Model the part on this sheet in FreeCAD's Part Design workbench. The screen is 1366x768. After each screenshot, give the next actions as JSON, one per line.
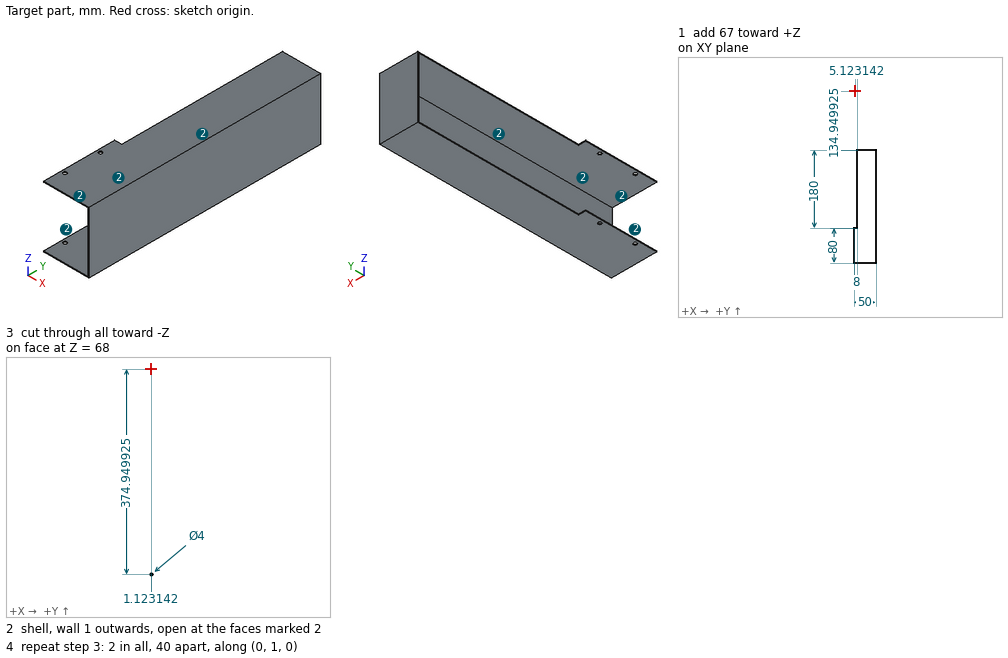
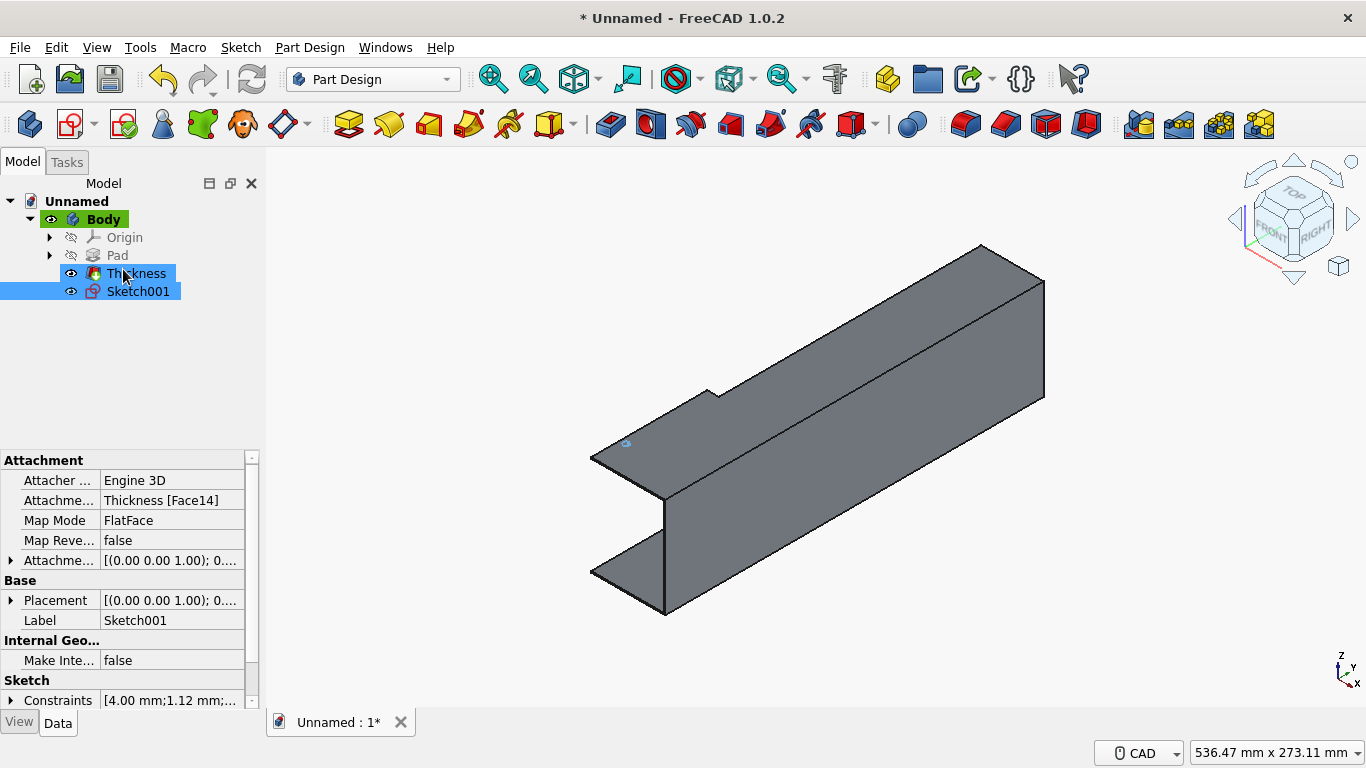
{"action": "left_click", "coordinate": [612, 124]}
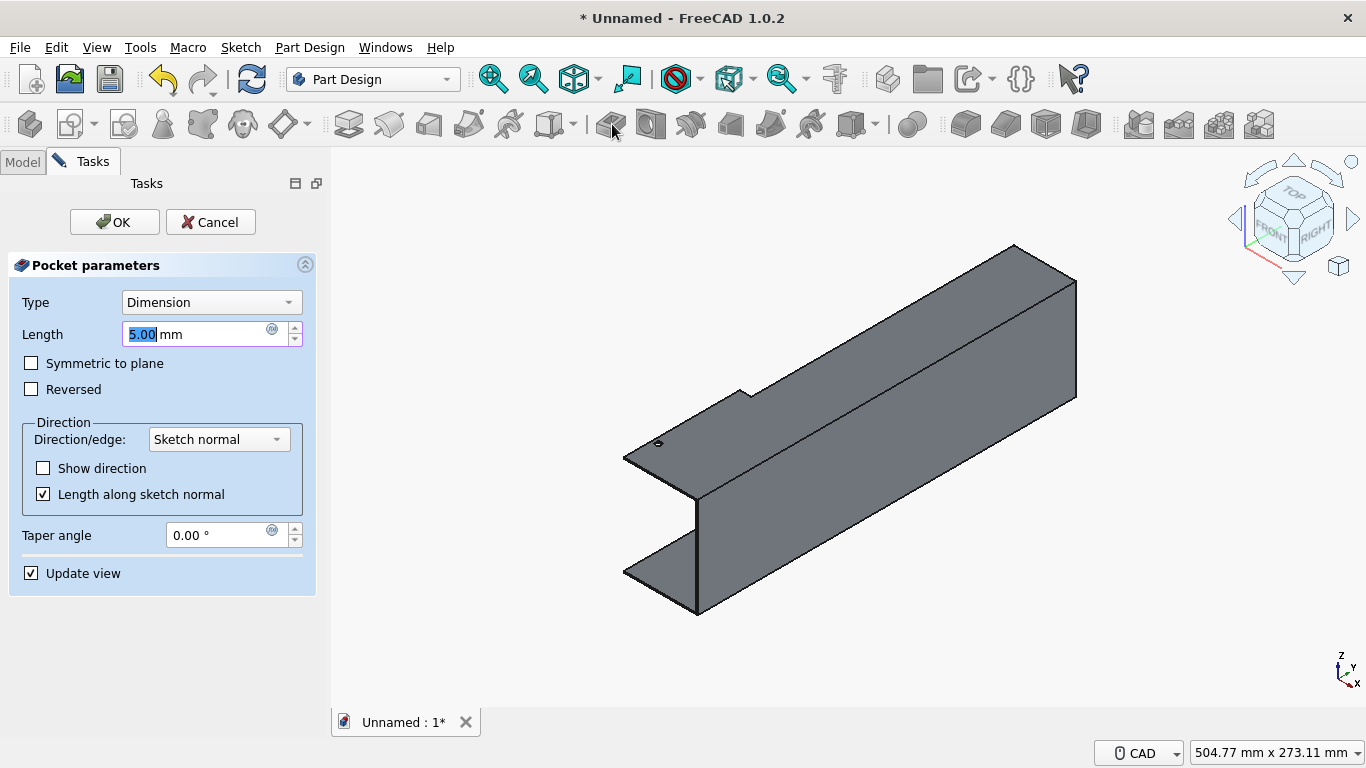
{"action": "left_click", "coordinate": [212, 302]}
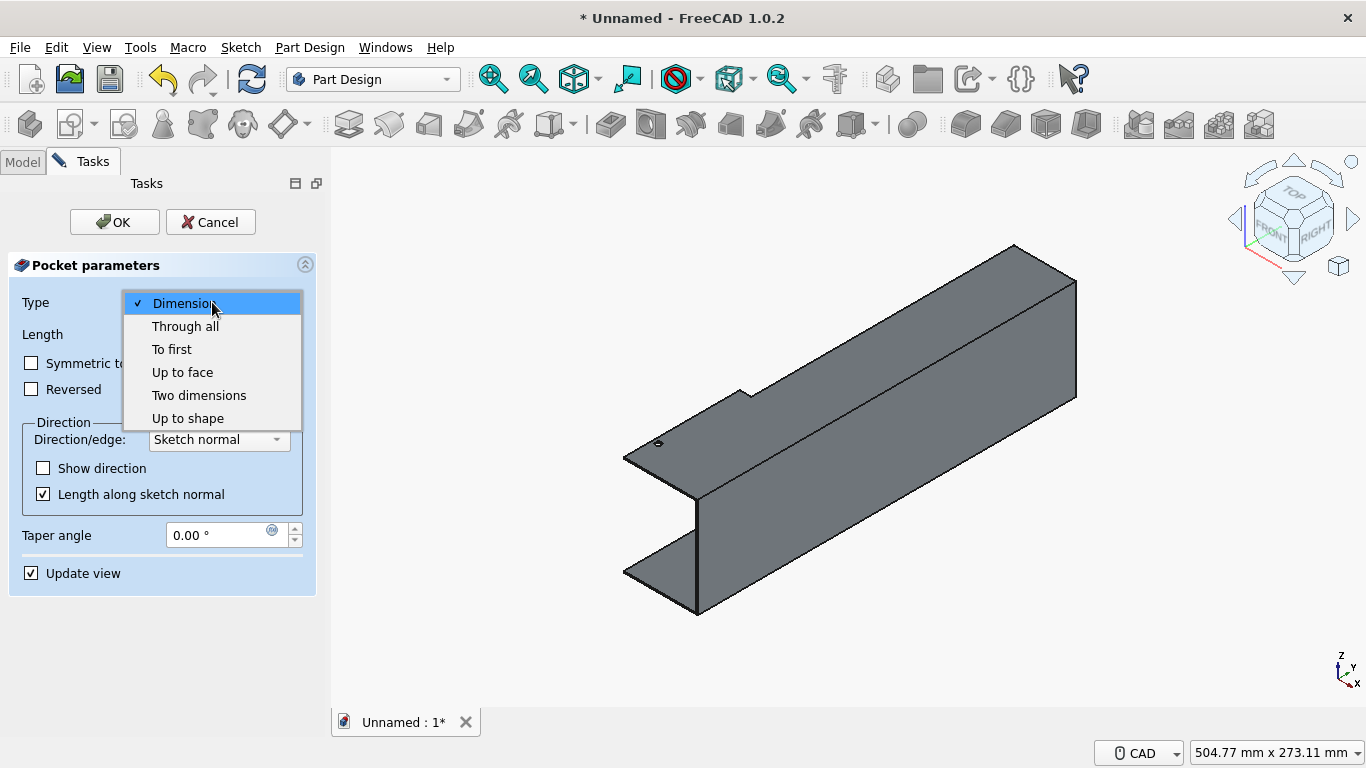
{"action": "left_click", "coordinate": [212, 326]}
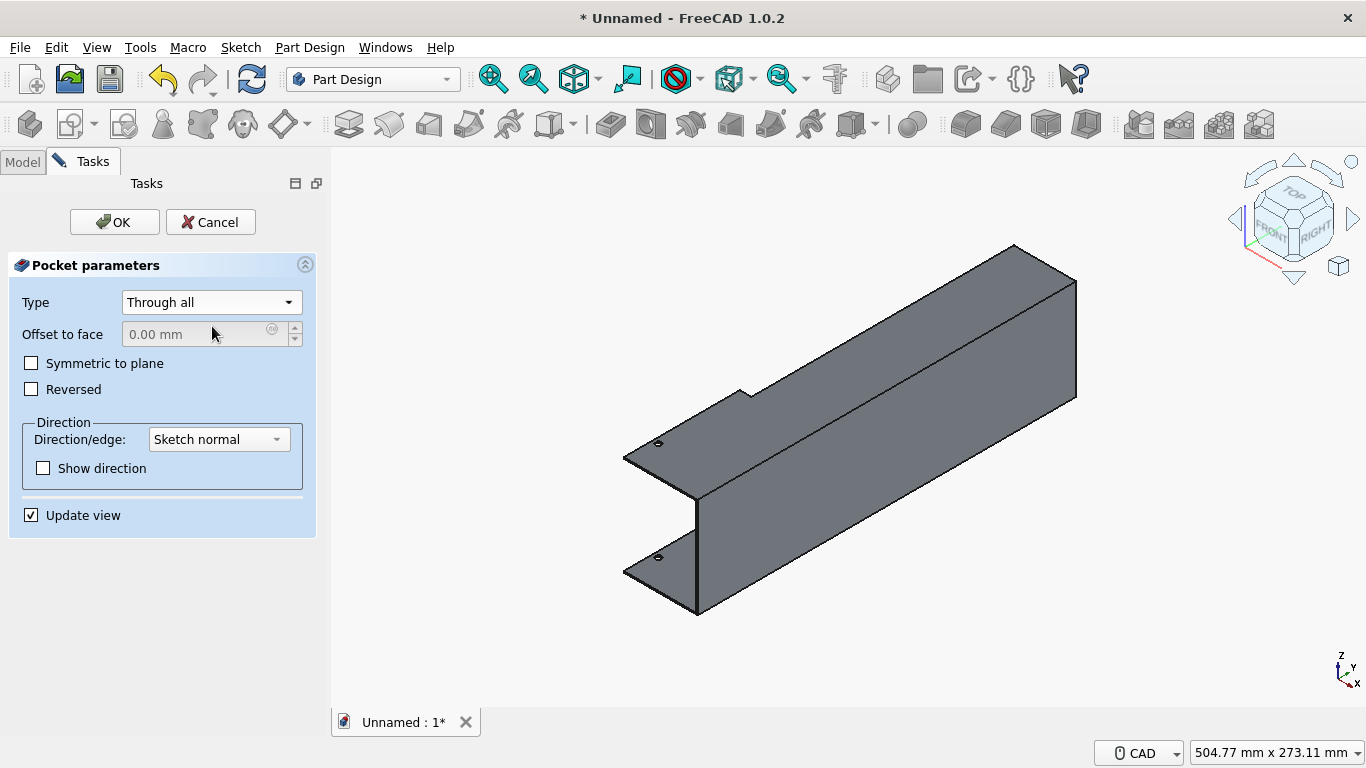
{"action": "left_click", "coordinate": [115, 222]}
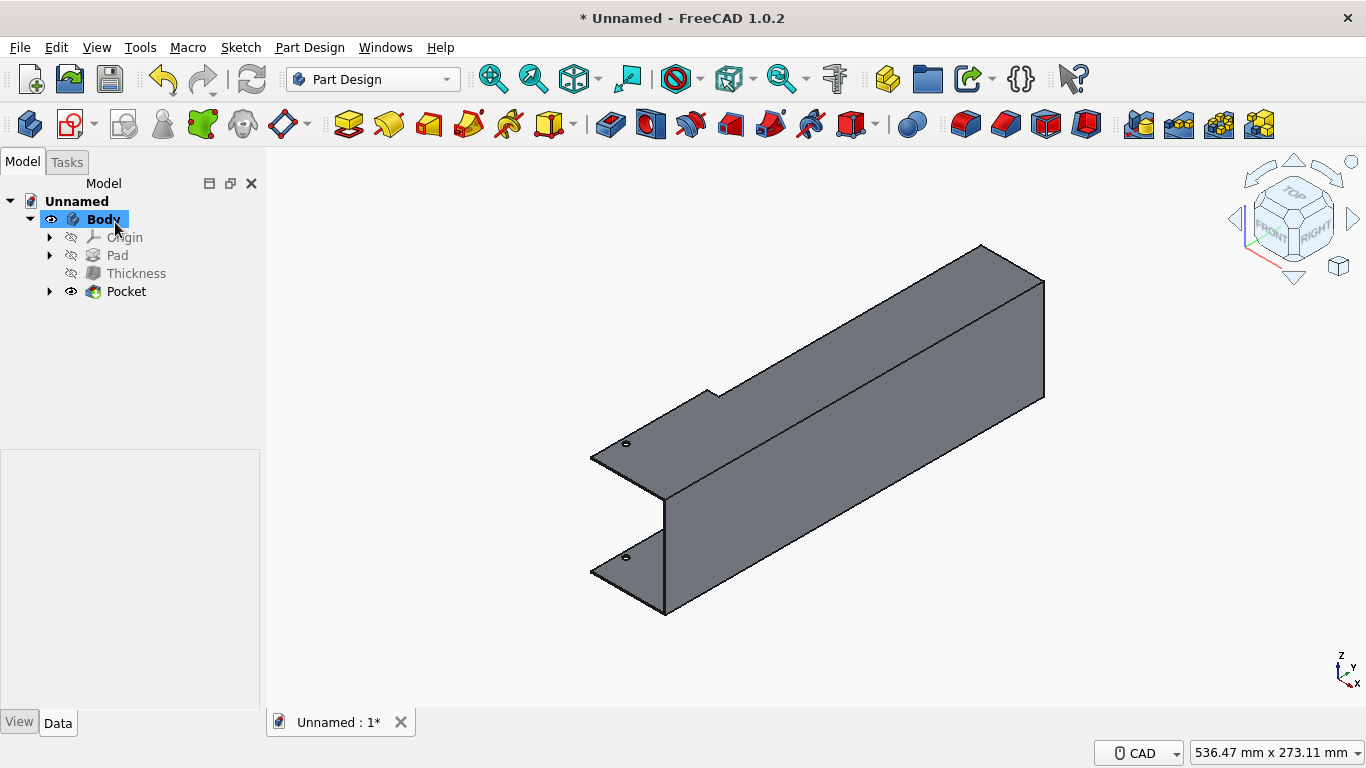
{"action": "left_click", "coordinate": [116, 291]}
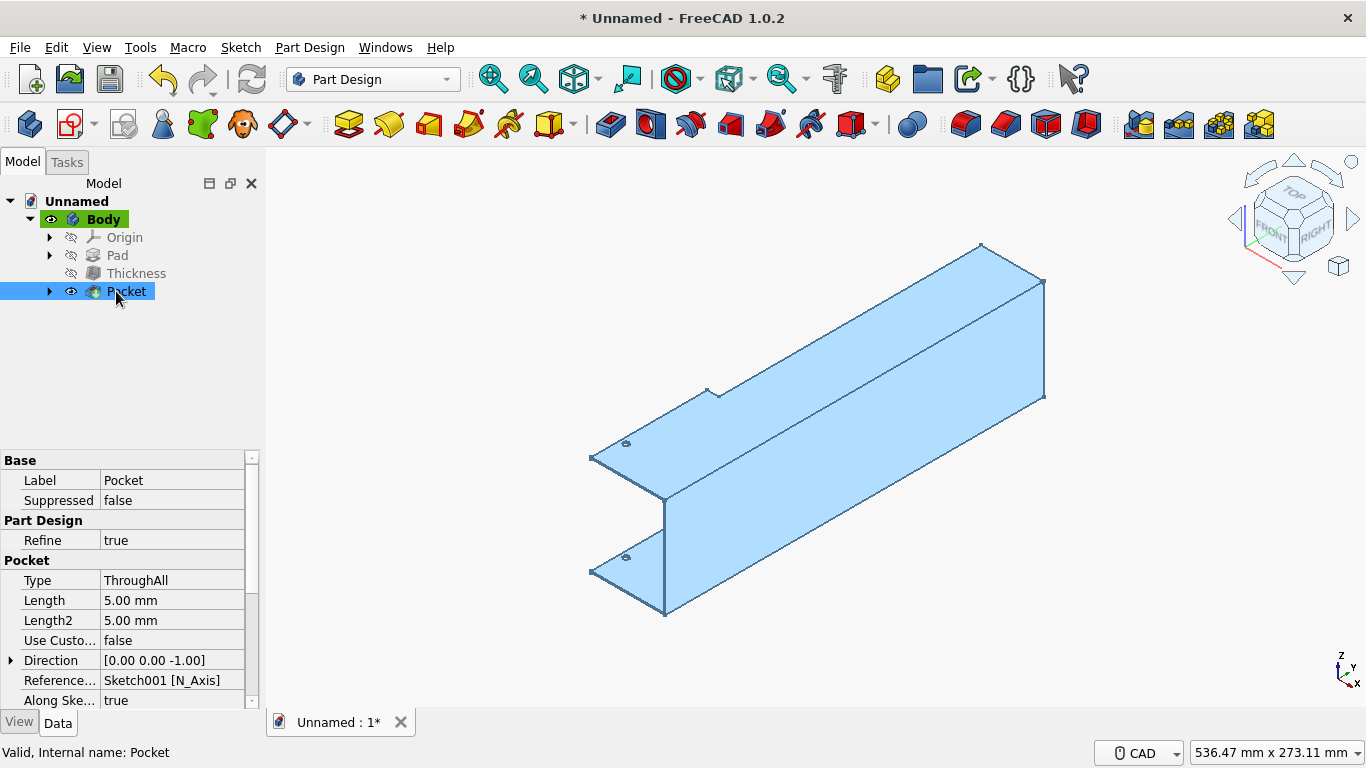
{"action": "left_click", "coordinate": [1180, 124]}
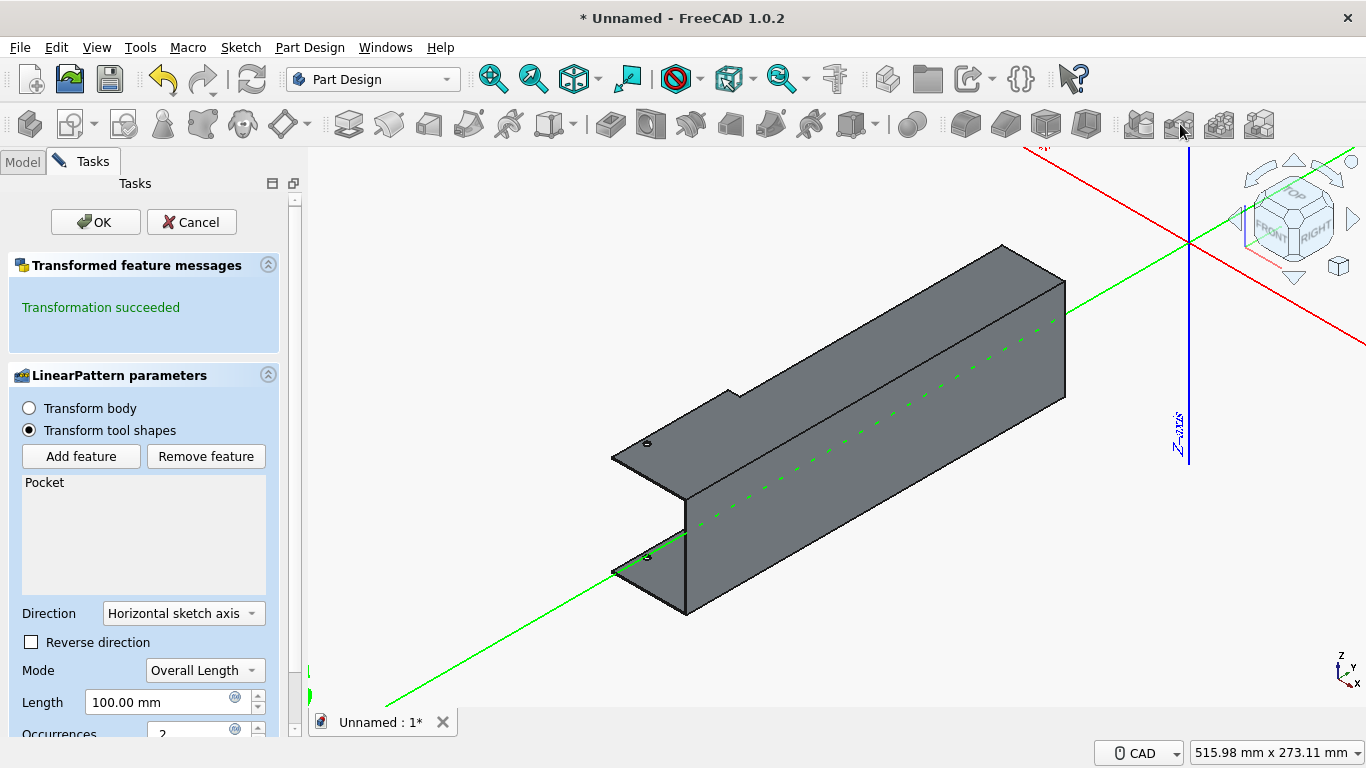
{"action": "left_click", "coordinate": [184, 614]}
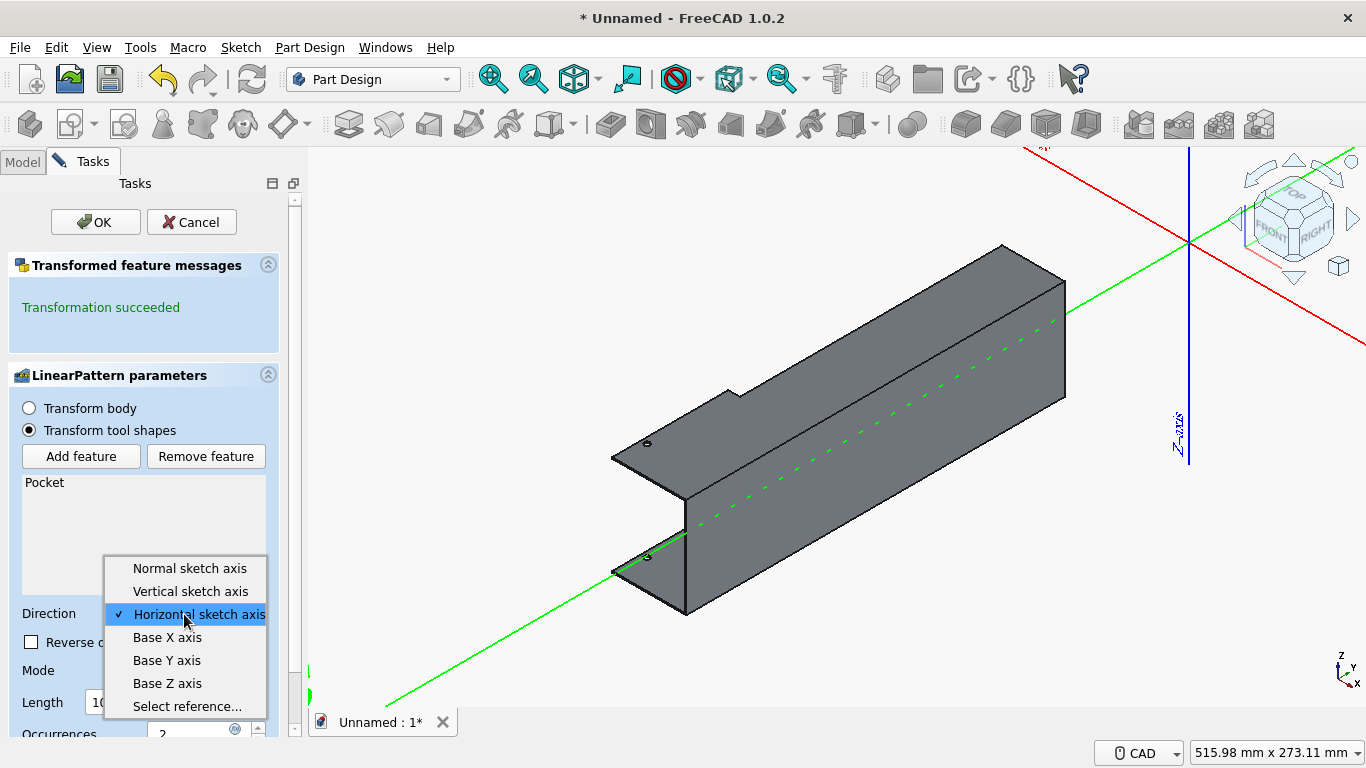
{"action": "left_click", "coordinate": [184, 660]}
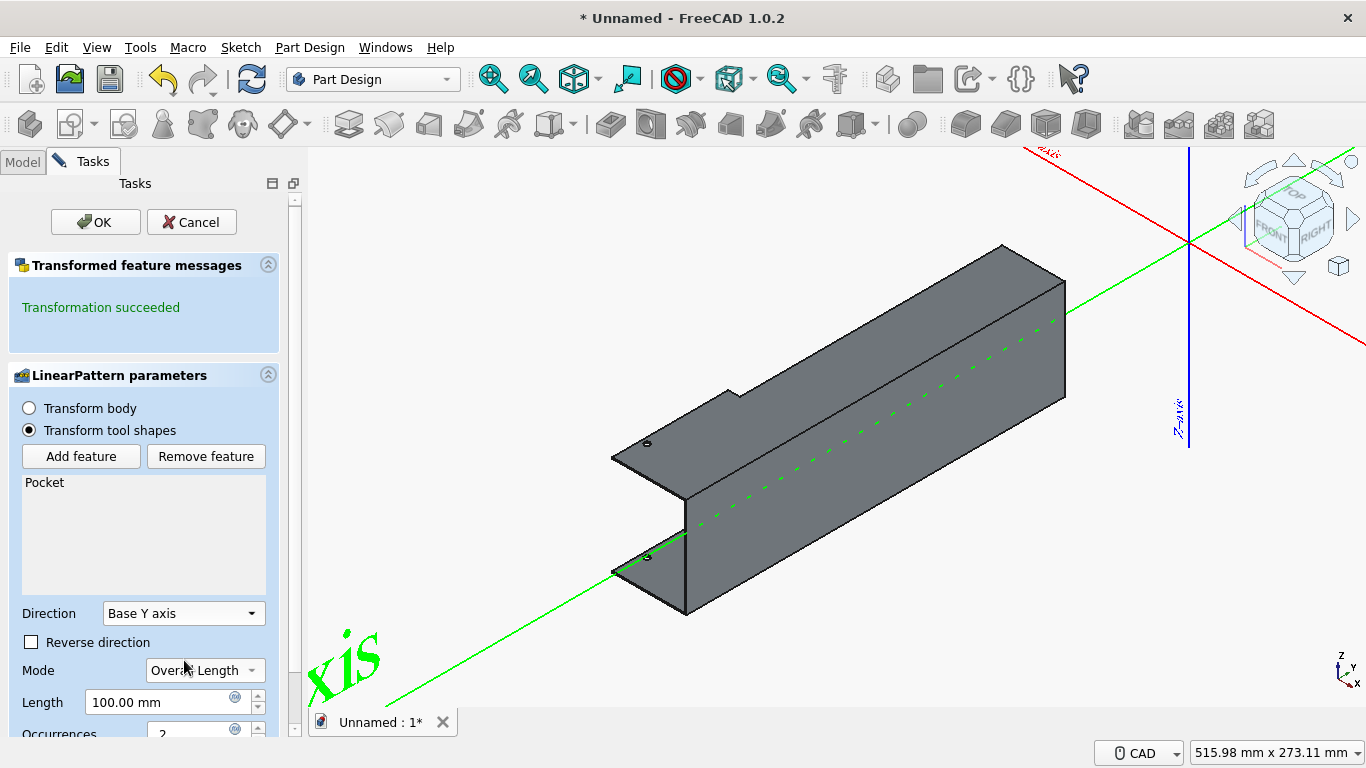
{"action": "left_click", "coordinate": [206, 670]}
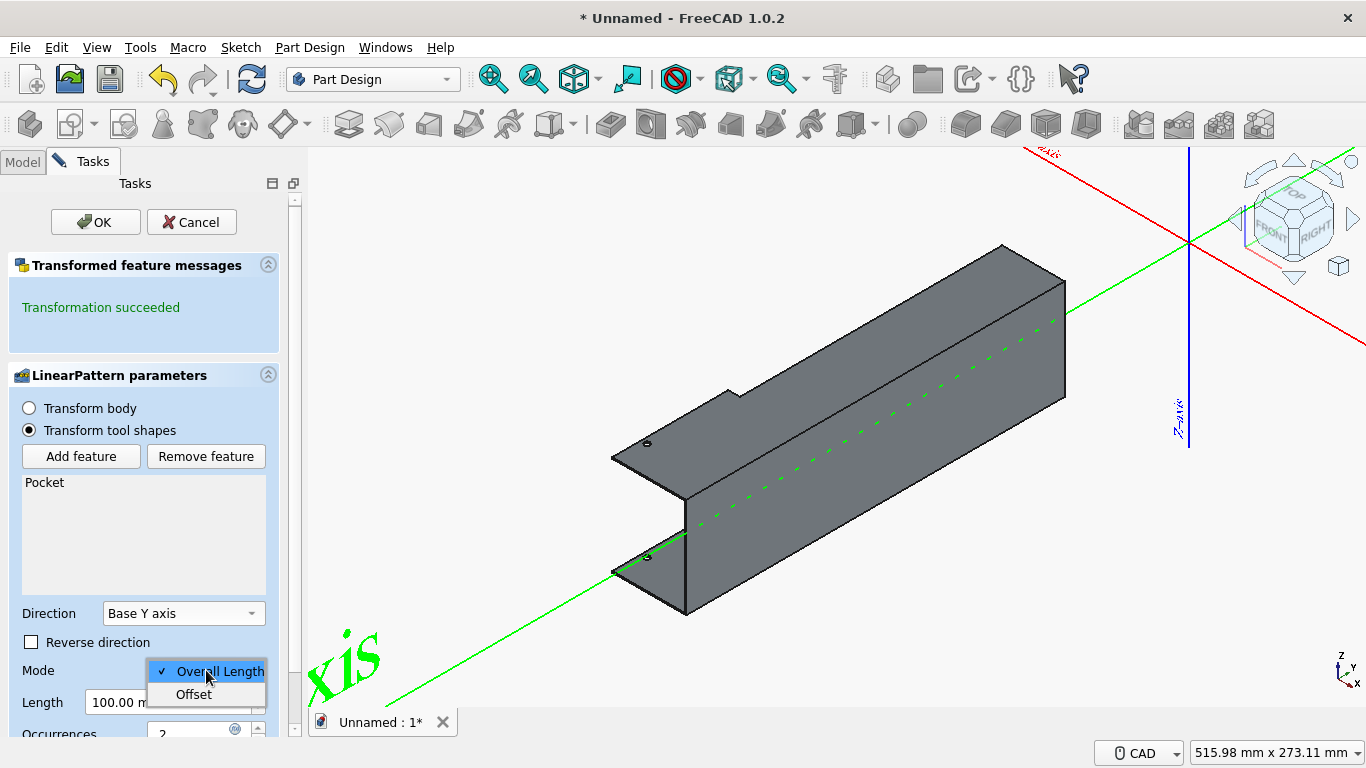
{"action": "left_click", "coordinate": [206, 694]}